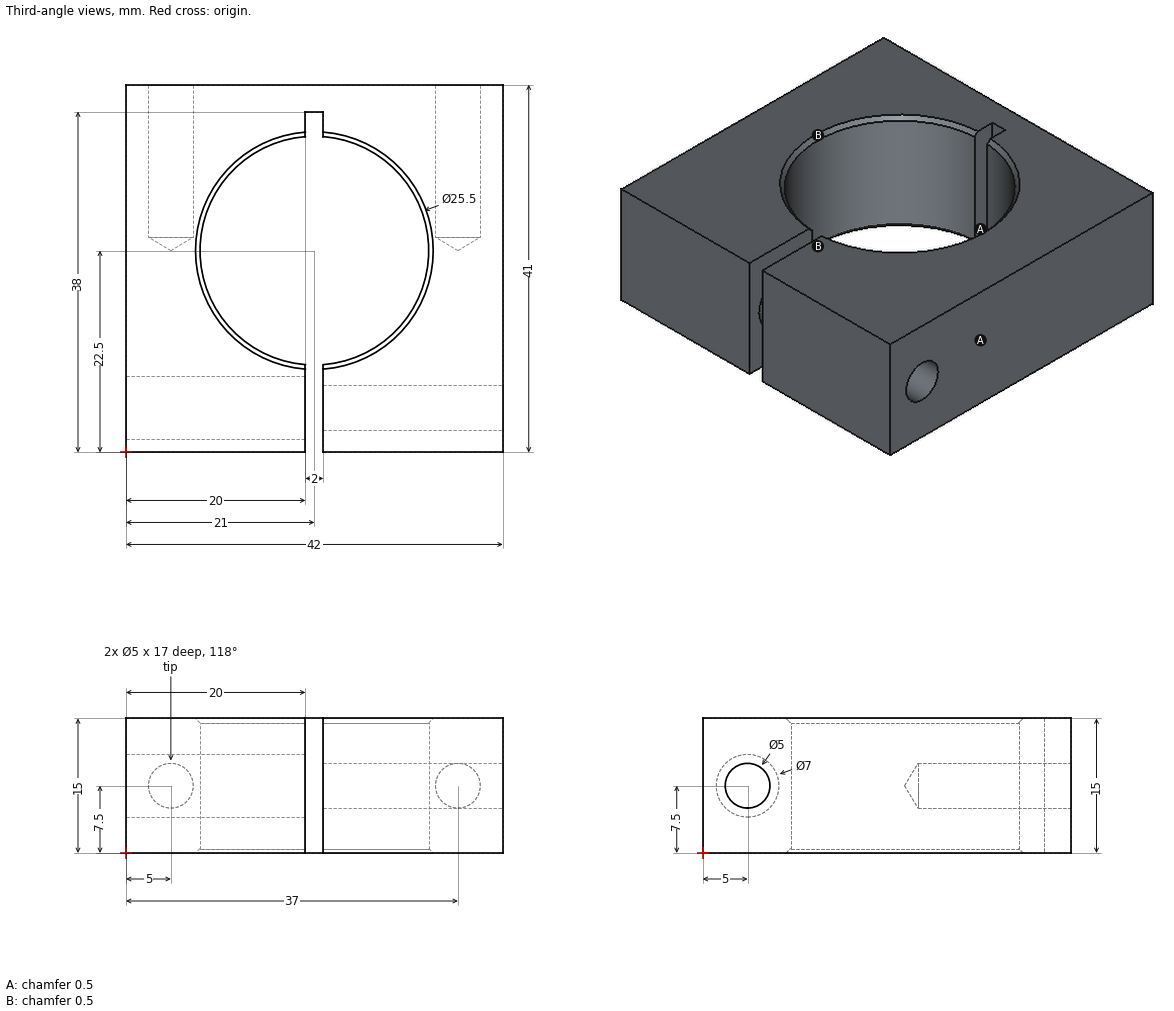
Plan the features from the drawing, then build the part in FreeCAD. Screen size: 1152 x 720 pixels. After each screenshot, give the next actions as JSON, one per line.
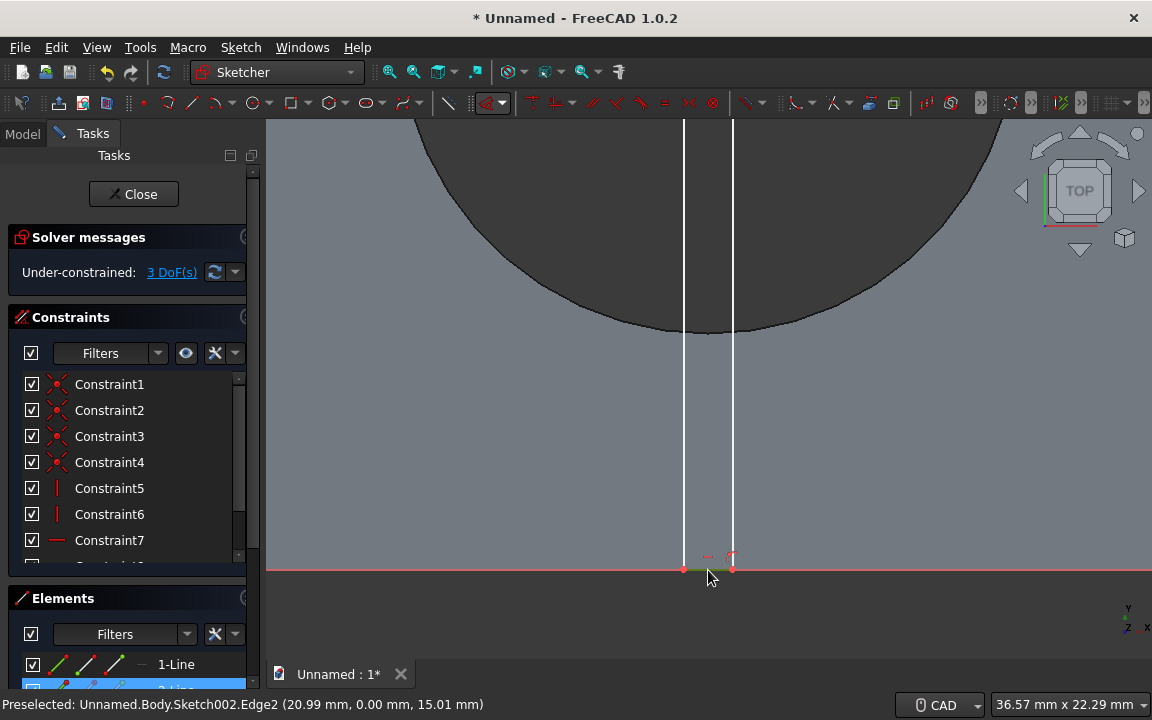
{"action": "left_click", "coordinate": [504, 104]}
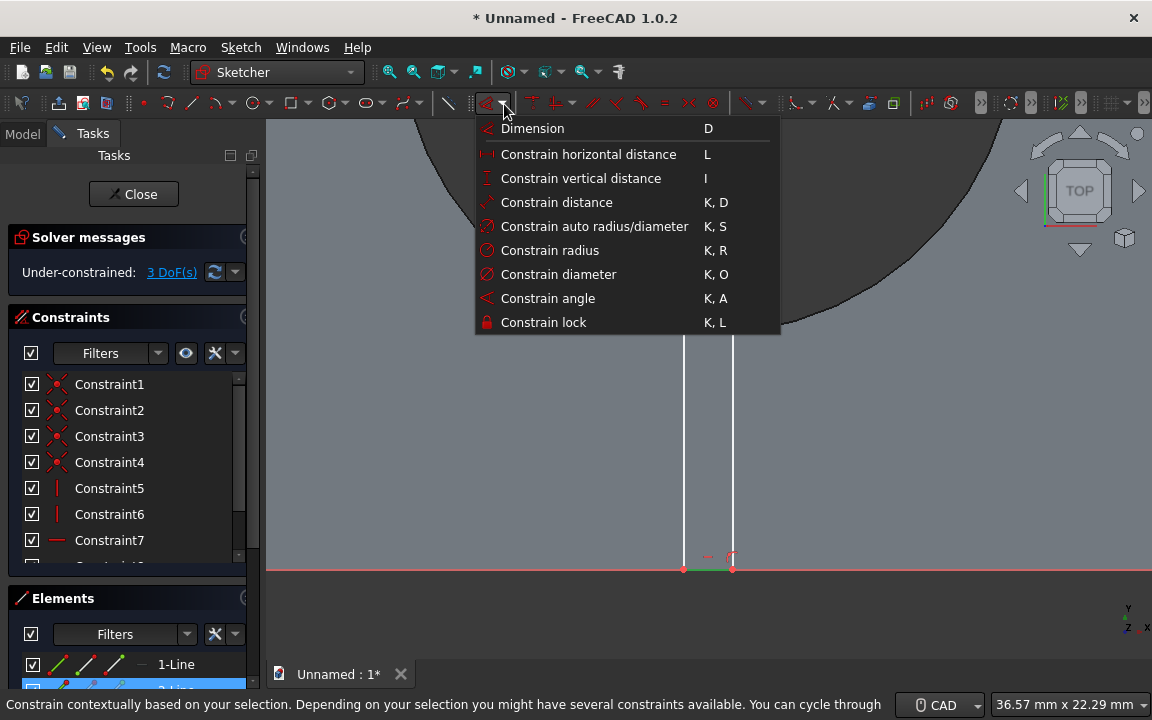
{"action": "left_click", "coordinate": [628, 154]}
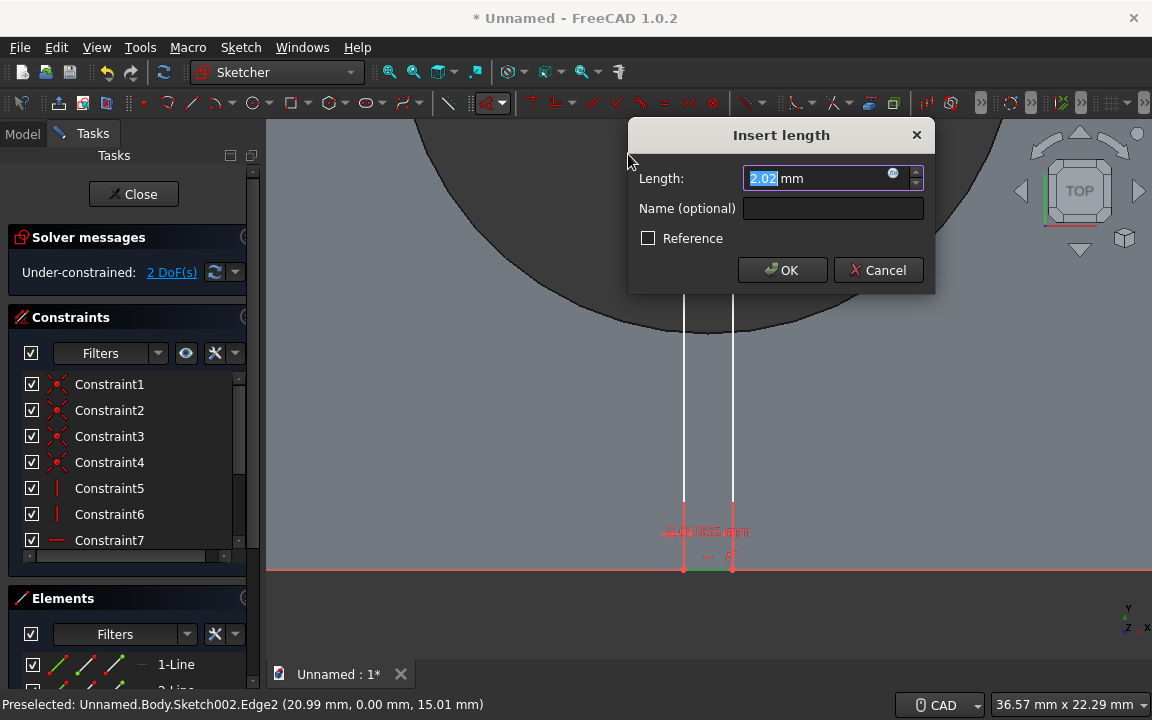
{"action": "type", "text": "2"}
{"action": "key", "text": "Return"}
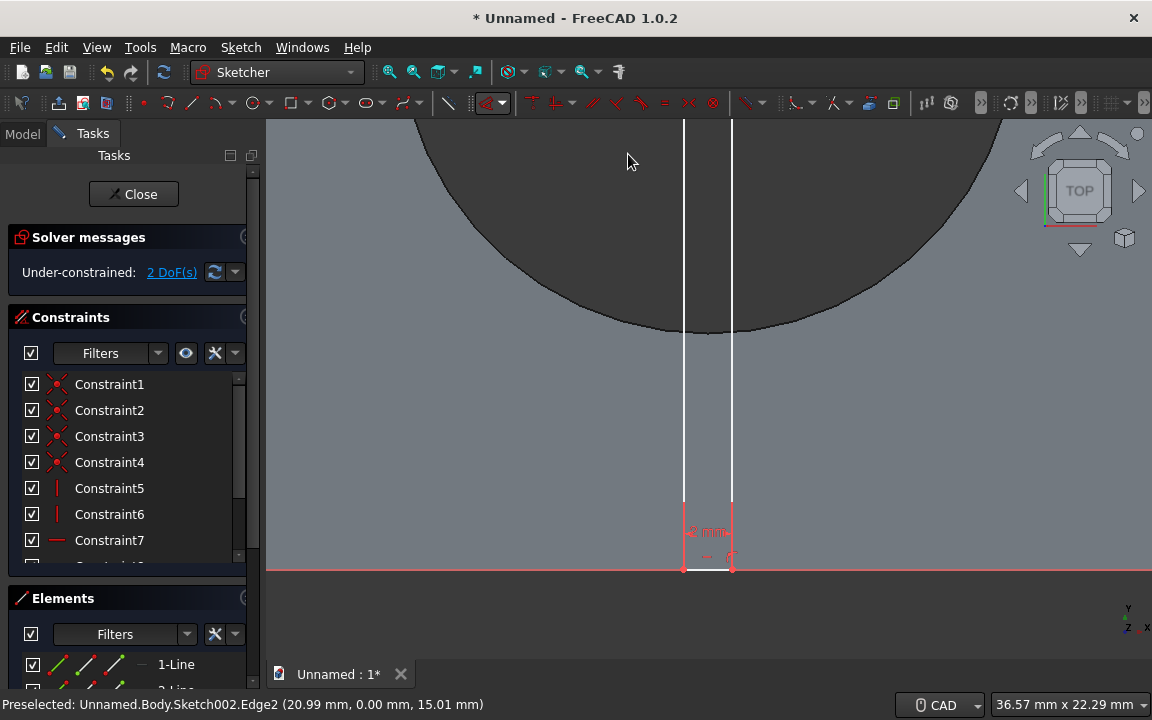
{"action": "left_click", "coordinate": [684, 294]}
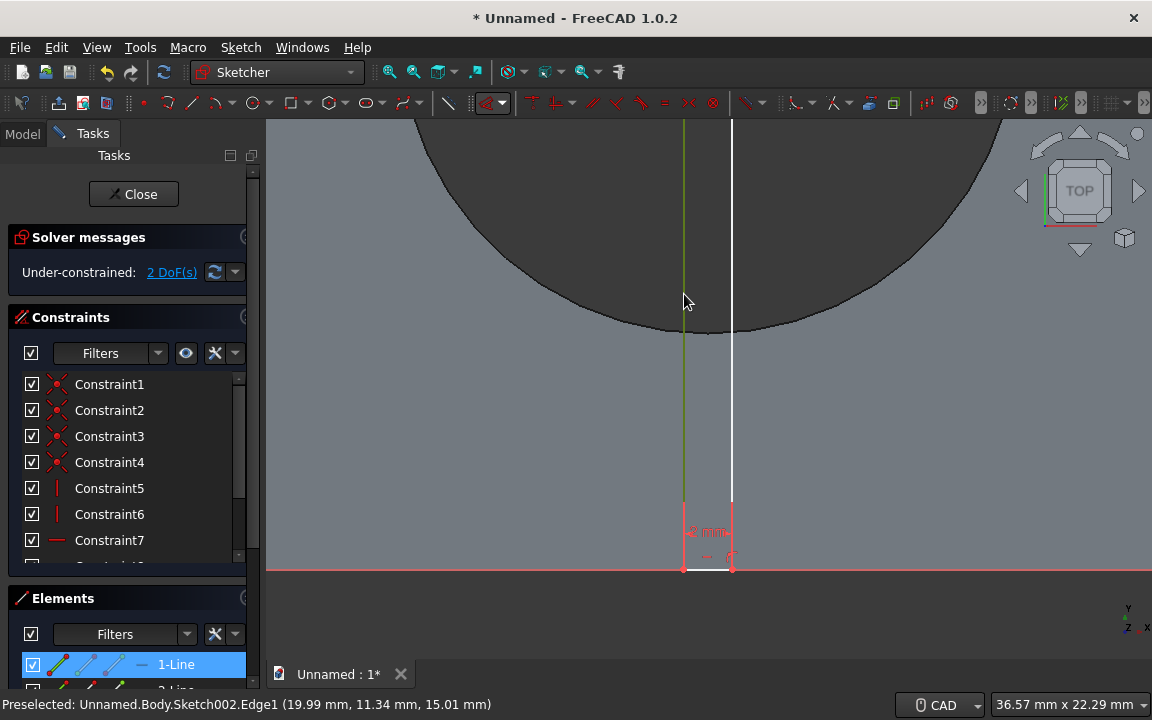
{"action": "left_click", "coordinate": [504, 104]}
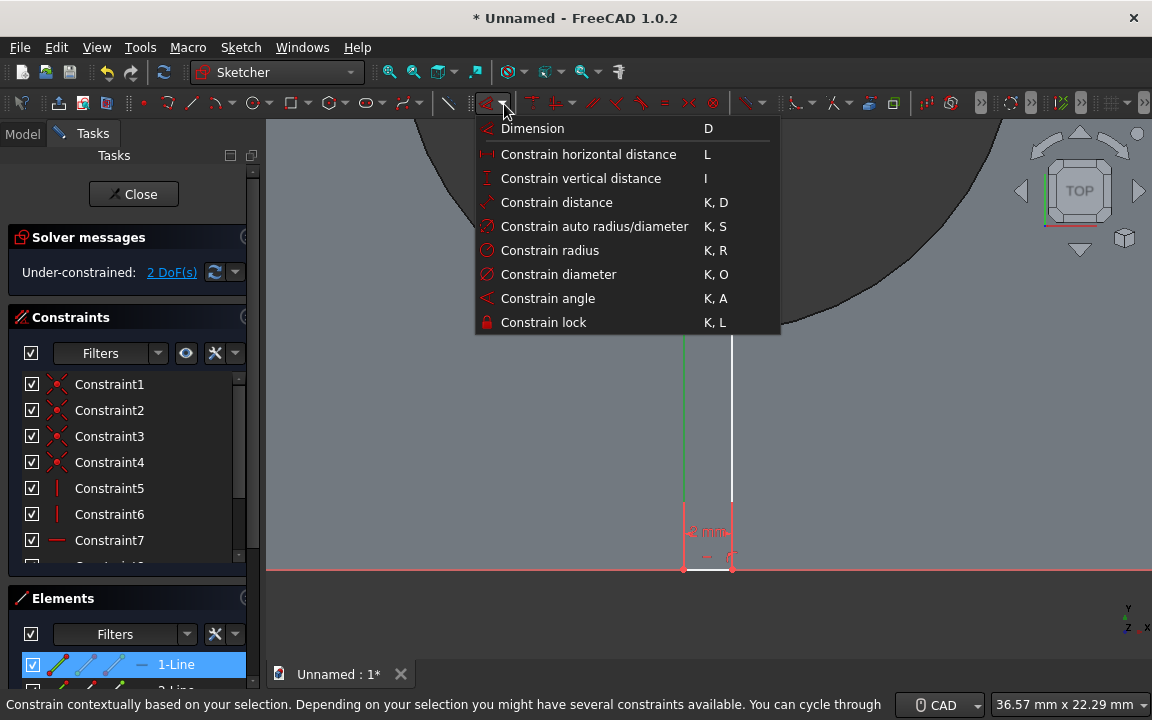
{"action": "left_click", "coordinate": [628, 178]}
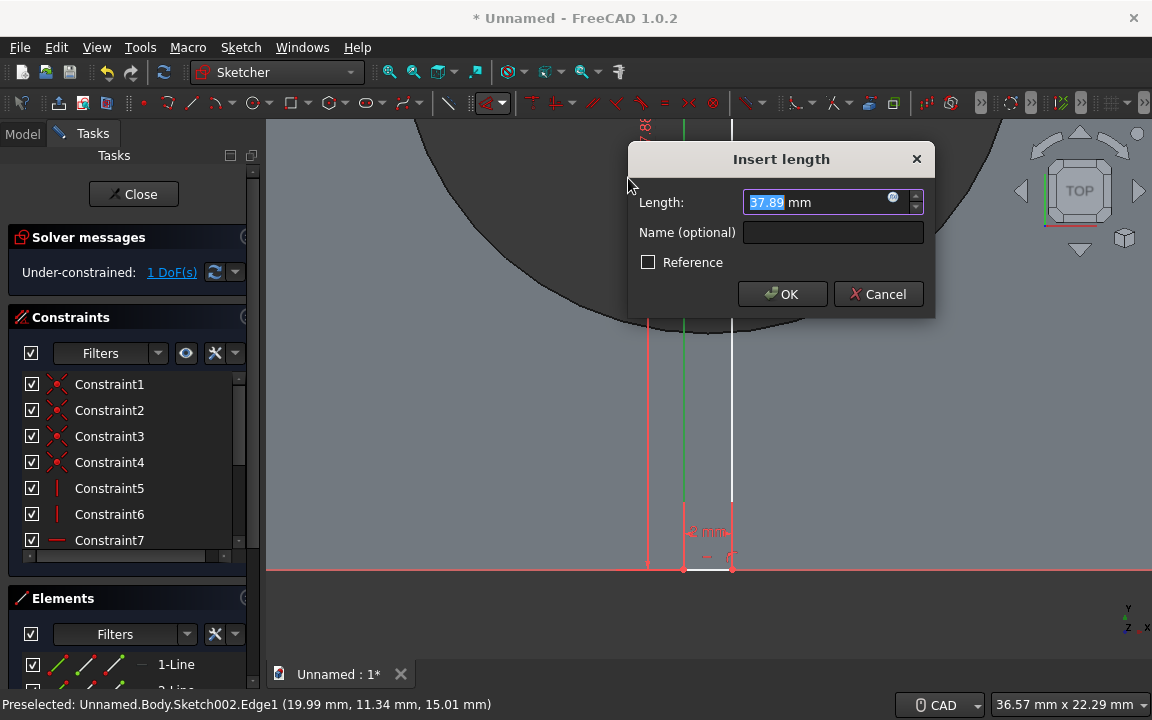
{"action": "type", "text": "38"}
{"action": "key", "text": "Return"}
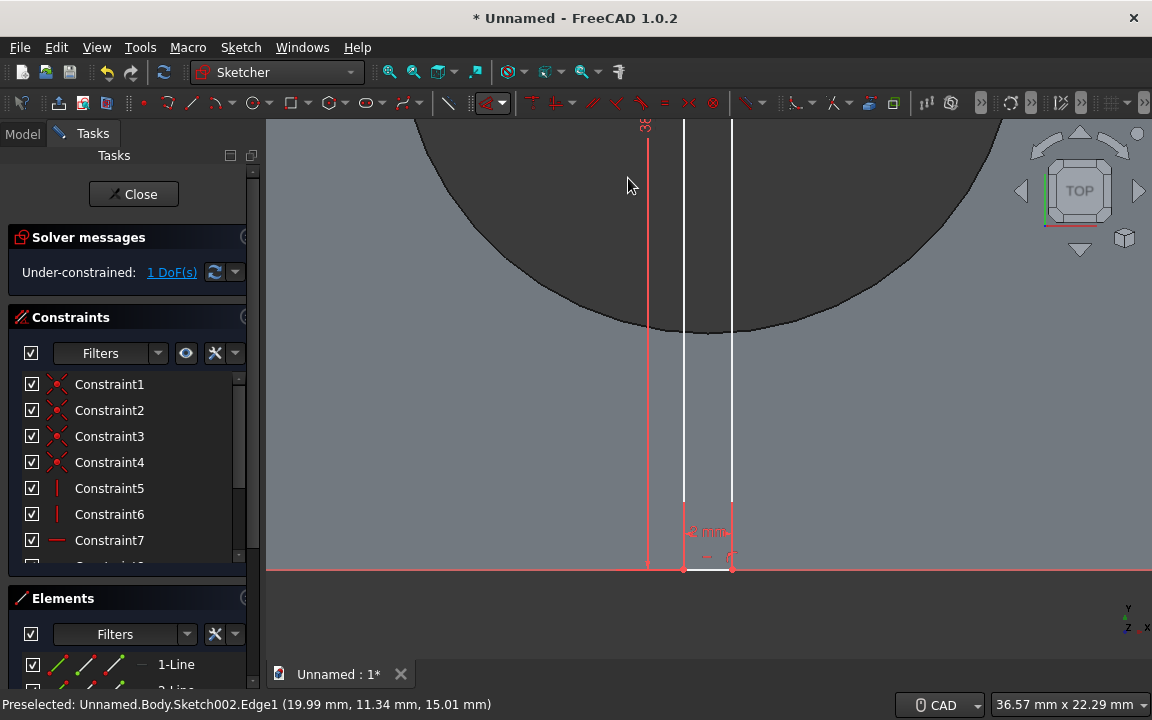
{"action": "scroll", "coordinate": [742, 552], "scroll_direction": "down", "scroll_amount": 5}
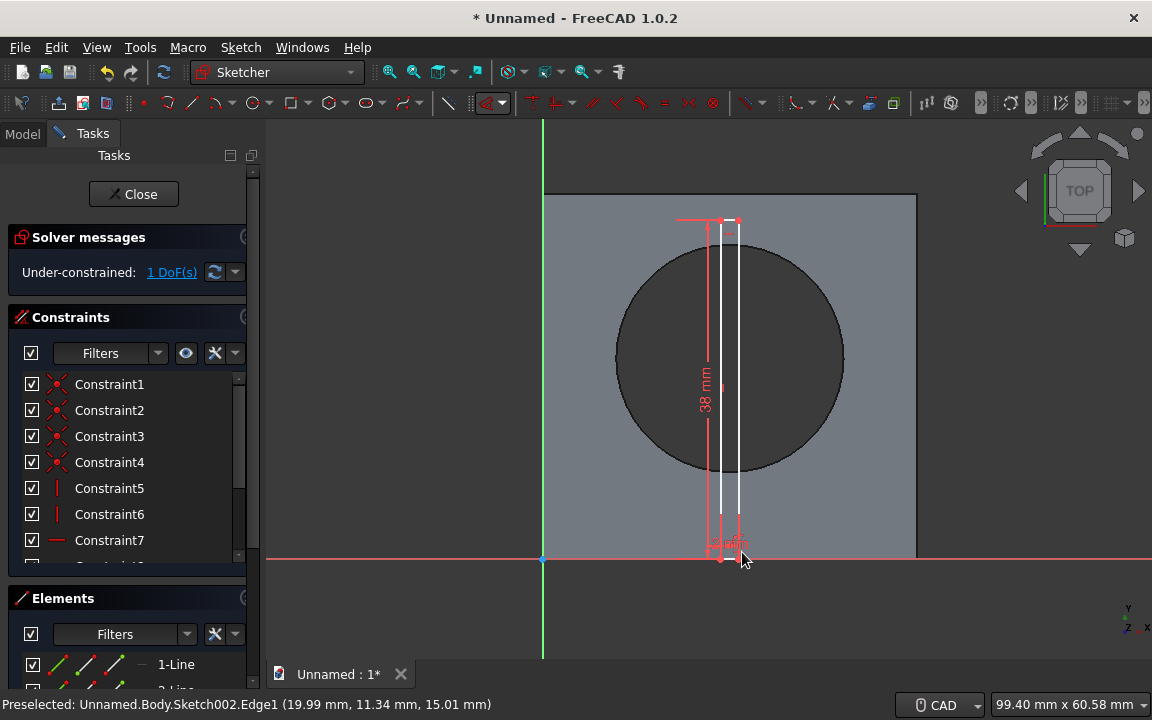
{"action": "left_click", "coordinate": [721, 220]}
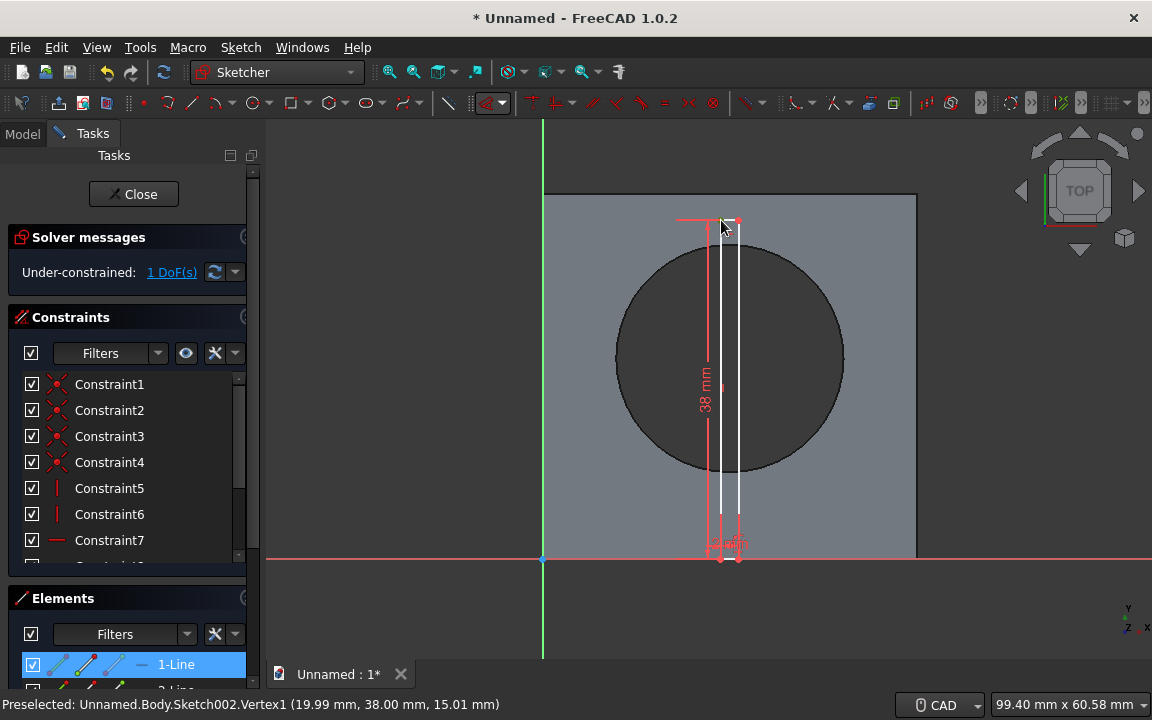
{"action": "key", "text": "l"}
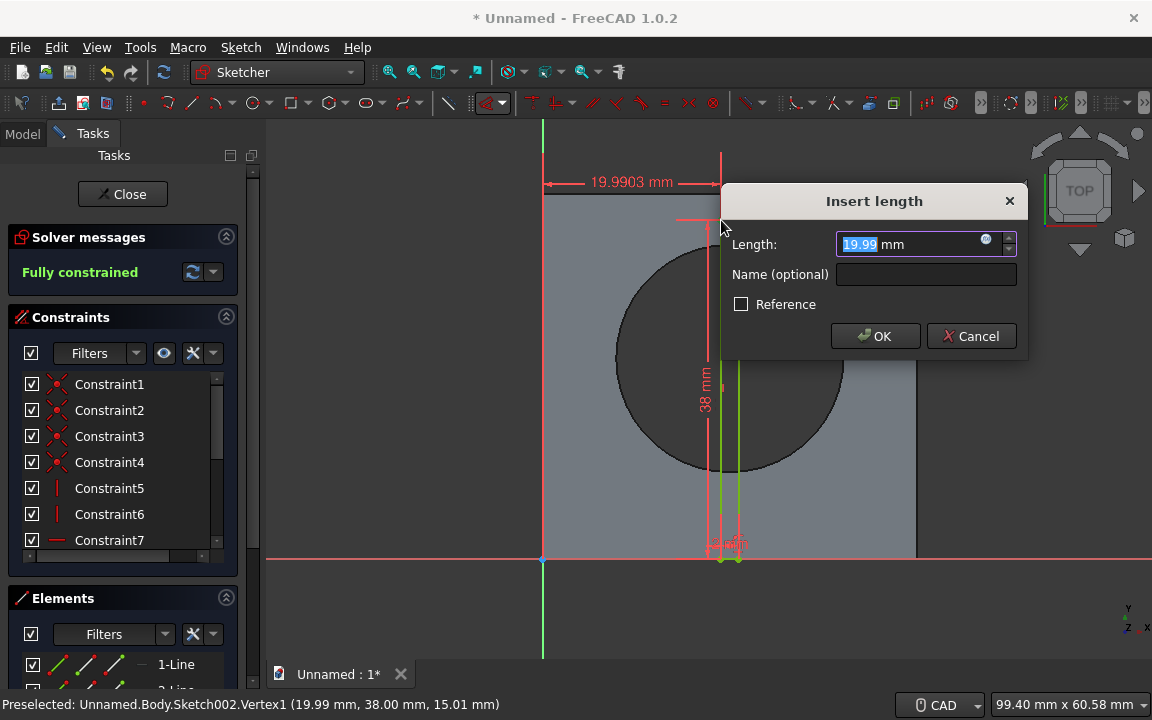
{"action": "type", "text": "20"}
{"action": "key", "text": "Return"}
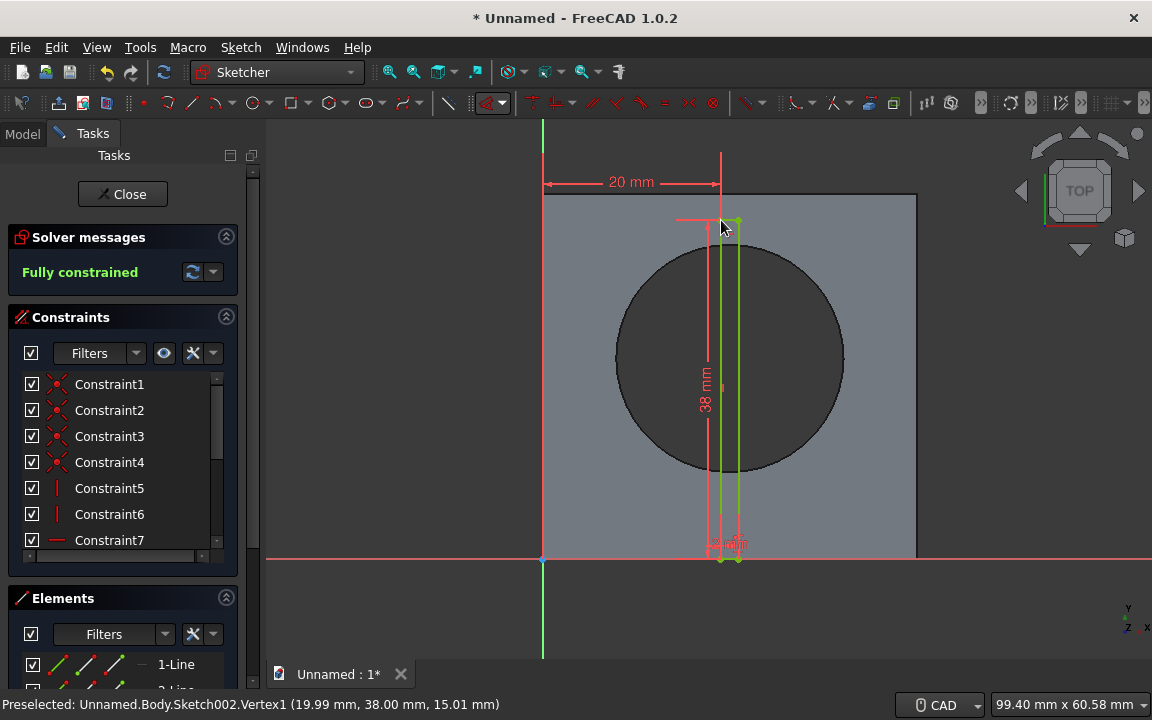
{"action": "left_click", "coordinate": [123, 194]}